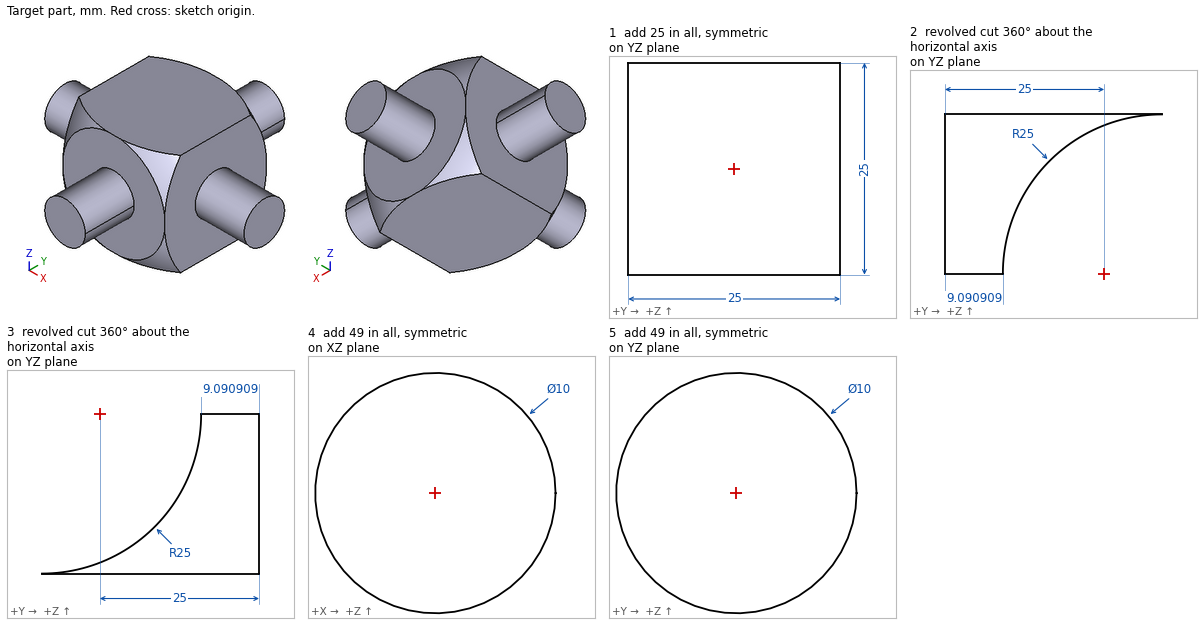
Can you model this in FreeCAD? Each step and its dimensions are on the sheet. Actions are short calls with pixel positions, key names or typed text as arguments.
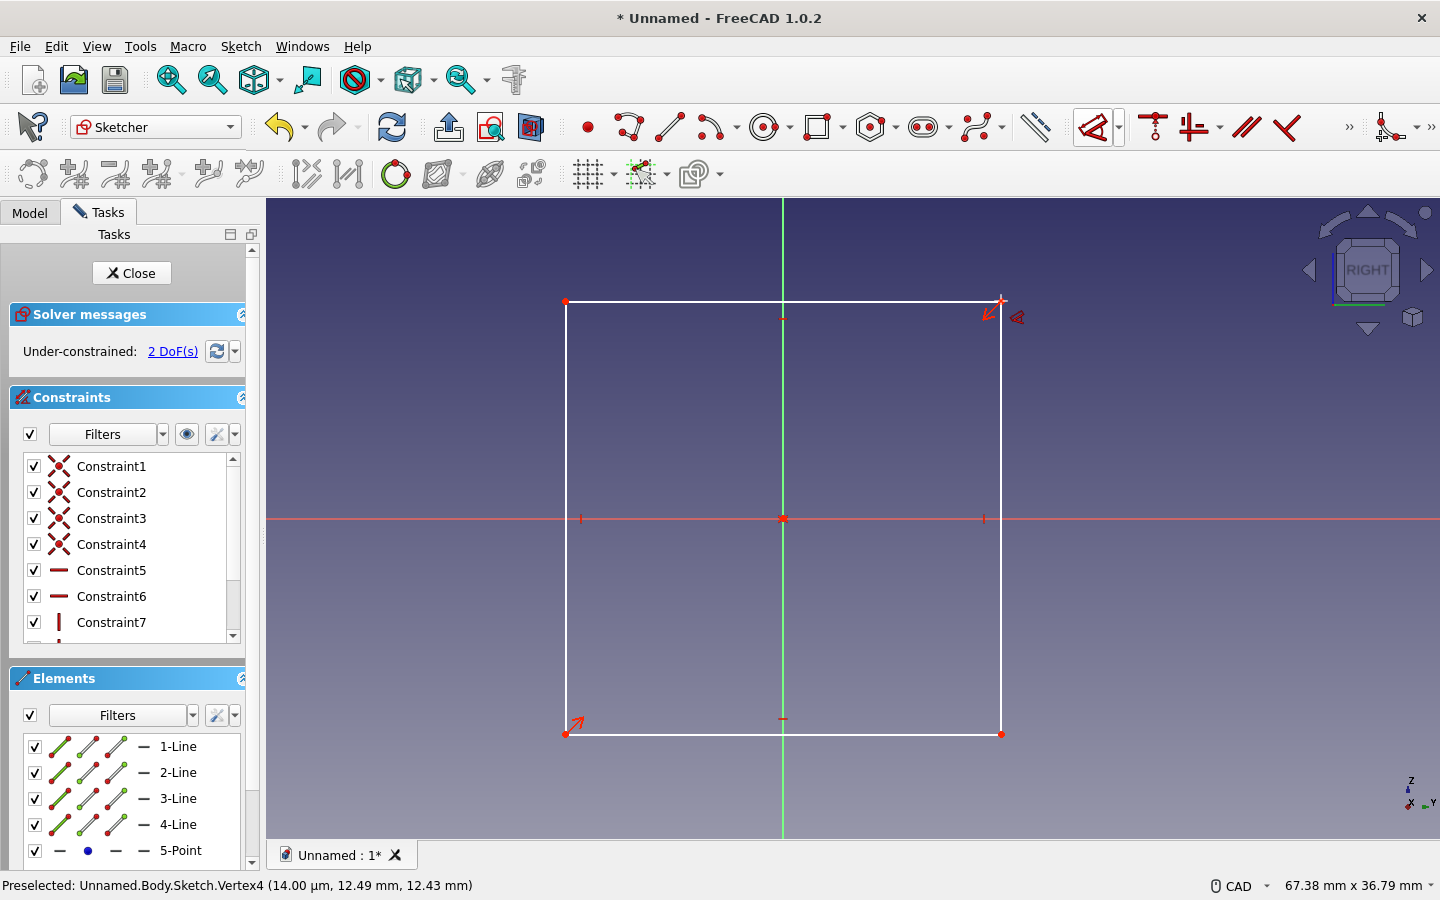
click(696, 735)
click(683, 769)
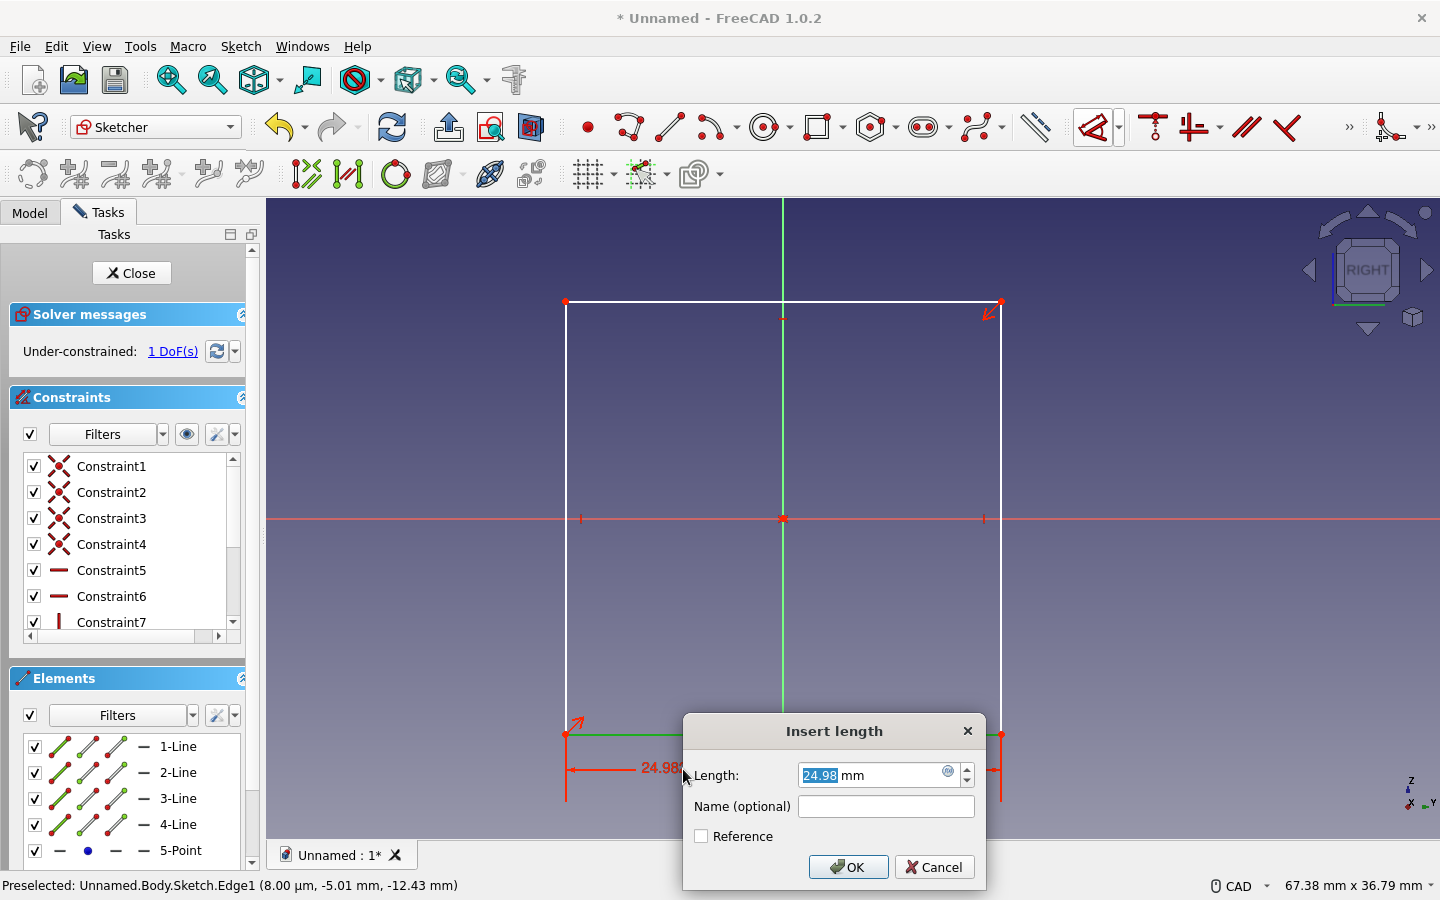
text(25)
key(Return)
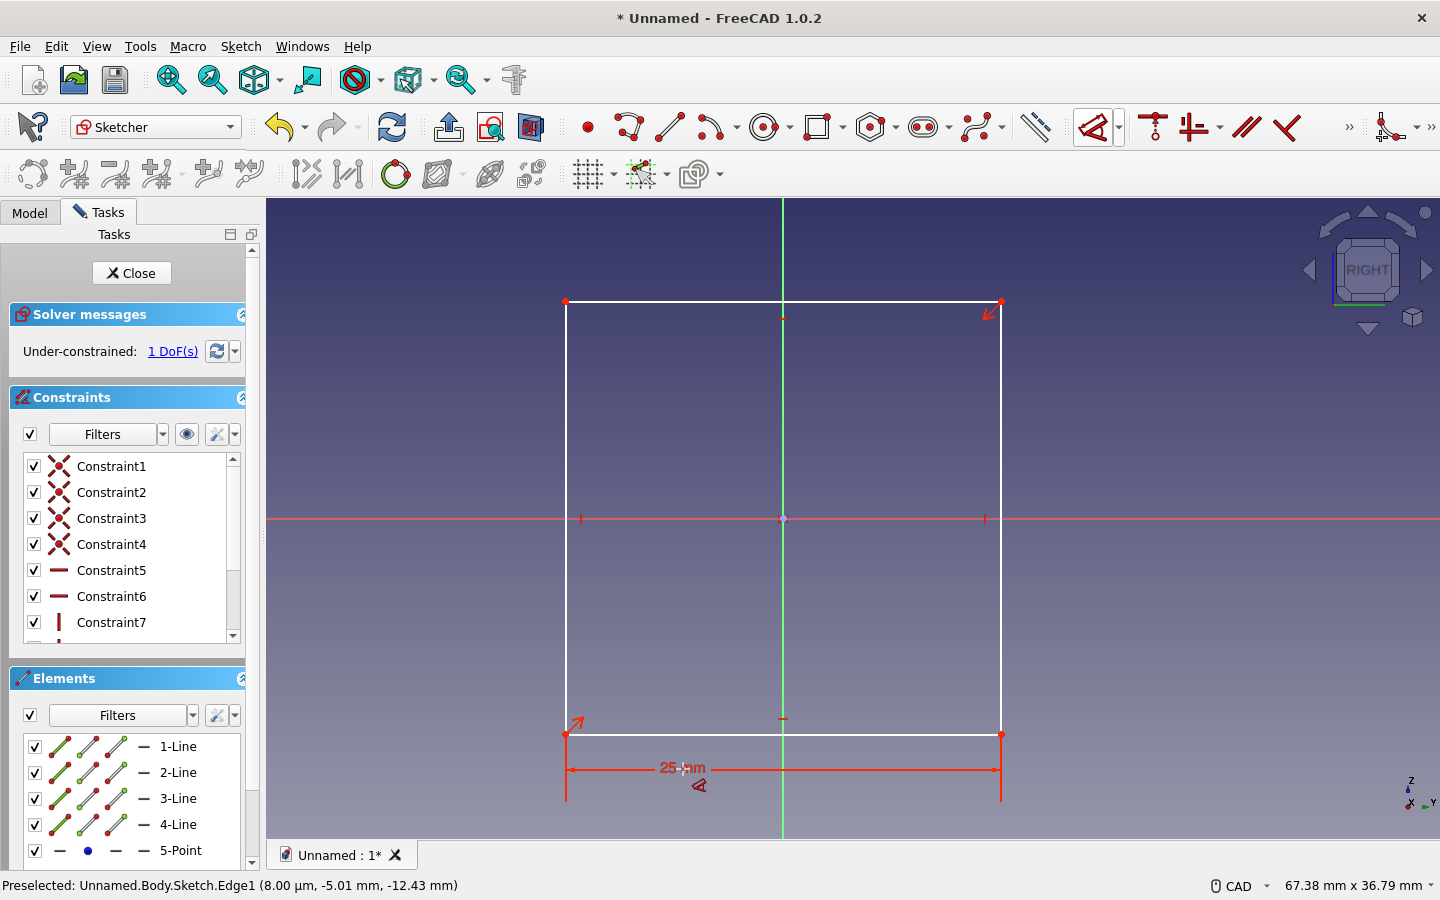
click(1001, 605)
click(1035, 419)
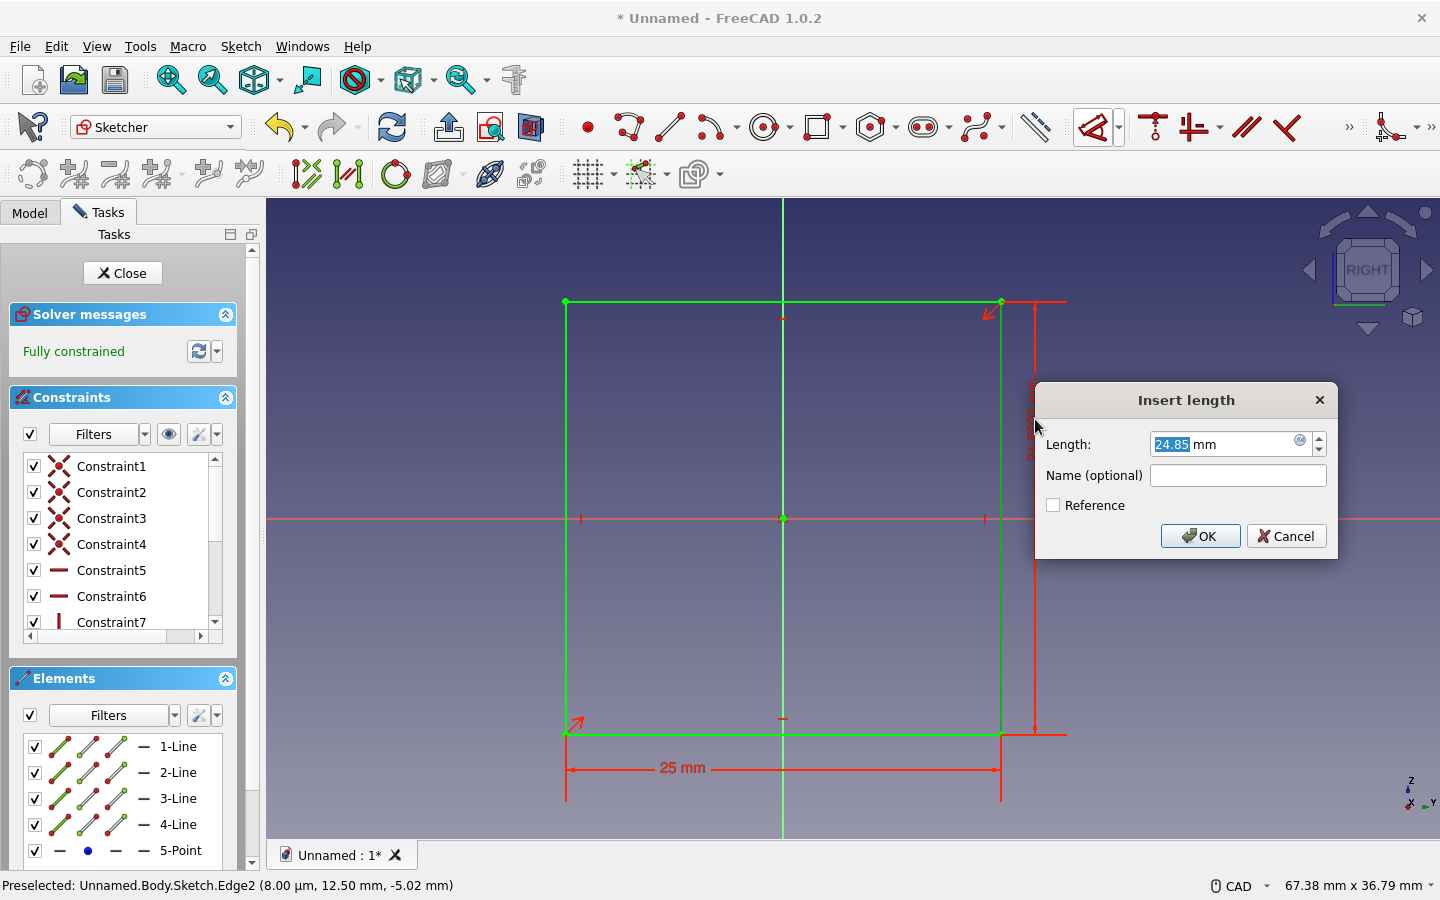
text(25)
key(Return)
key(Escape)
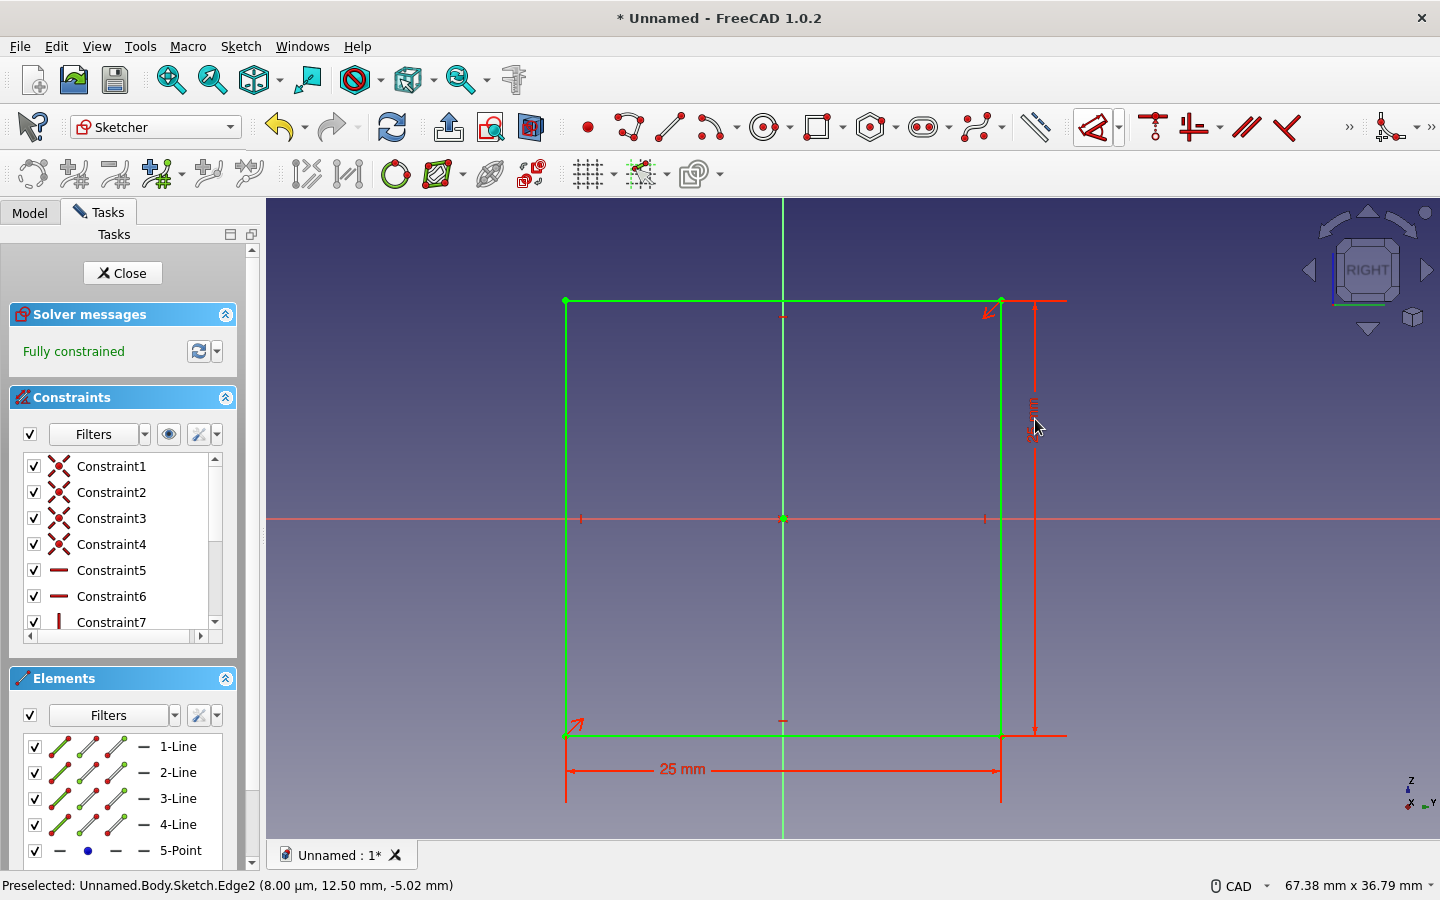
click(123, 273)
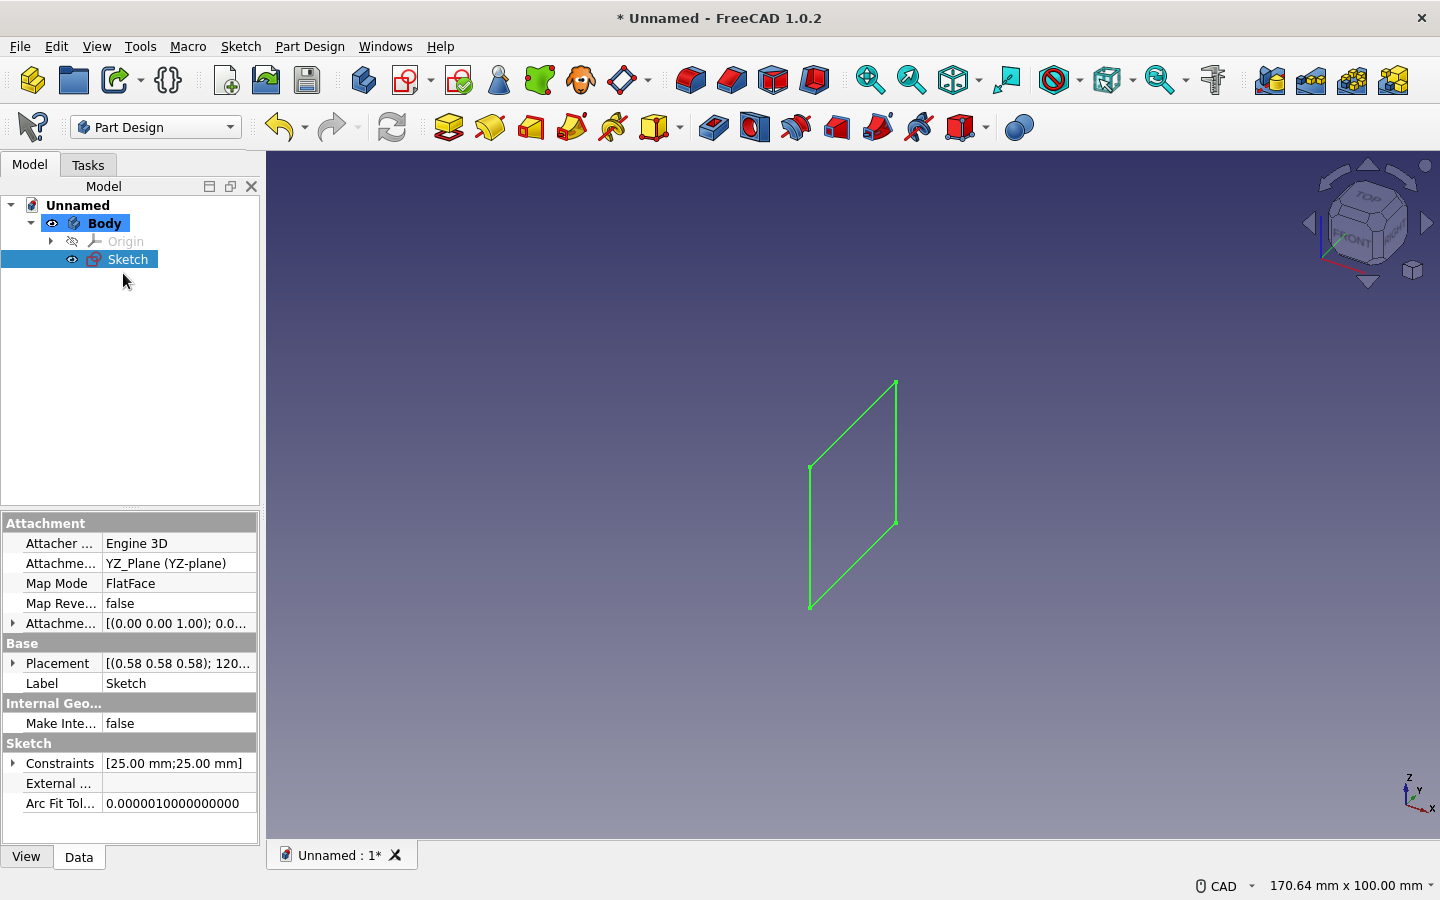
click(449, 128)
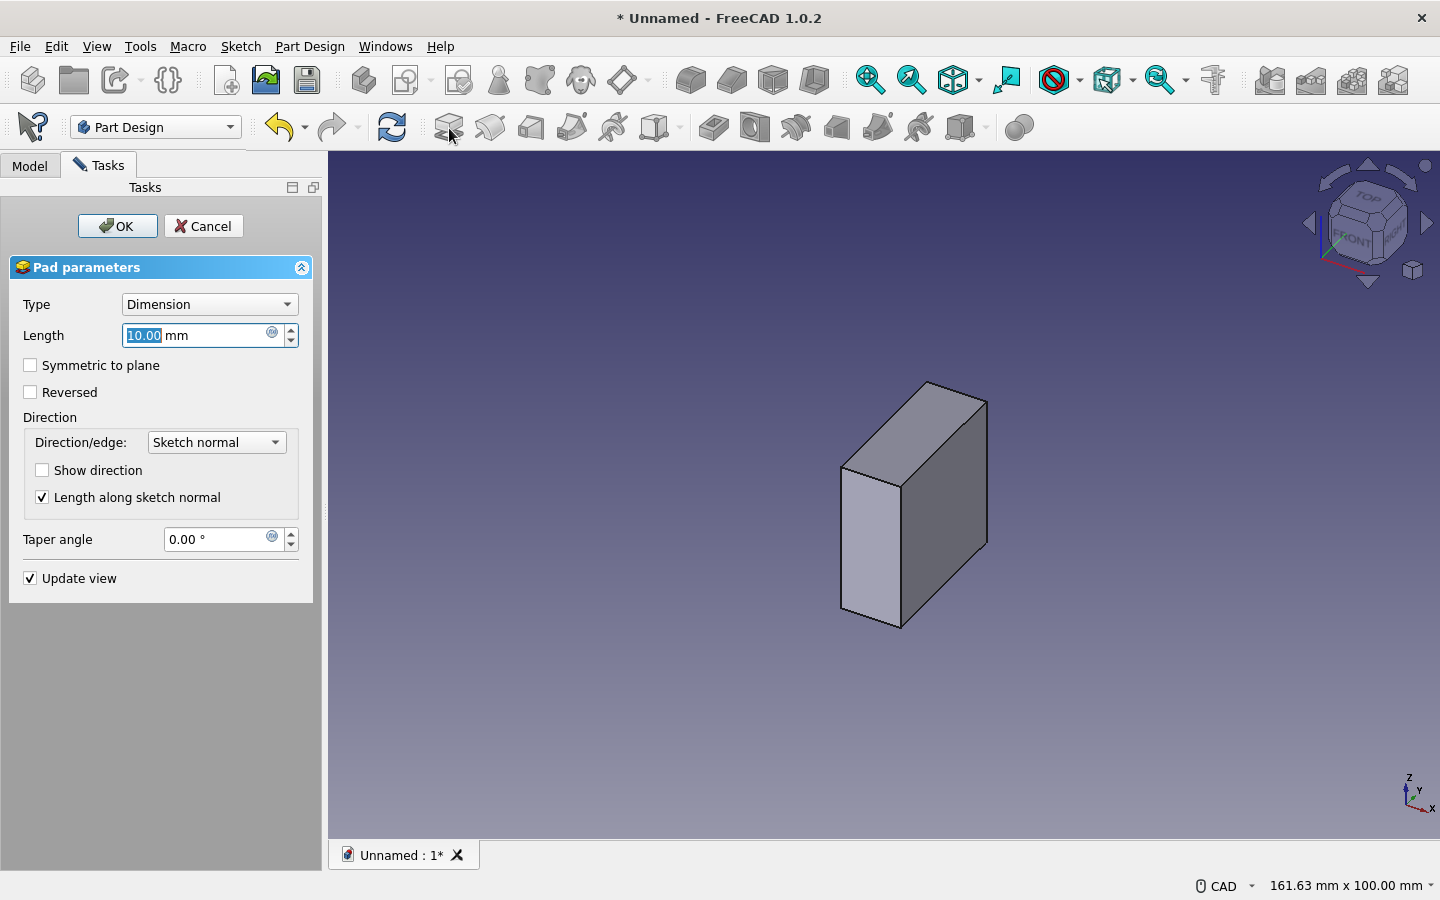
text(25)
key(Tab)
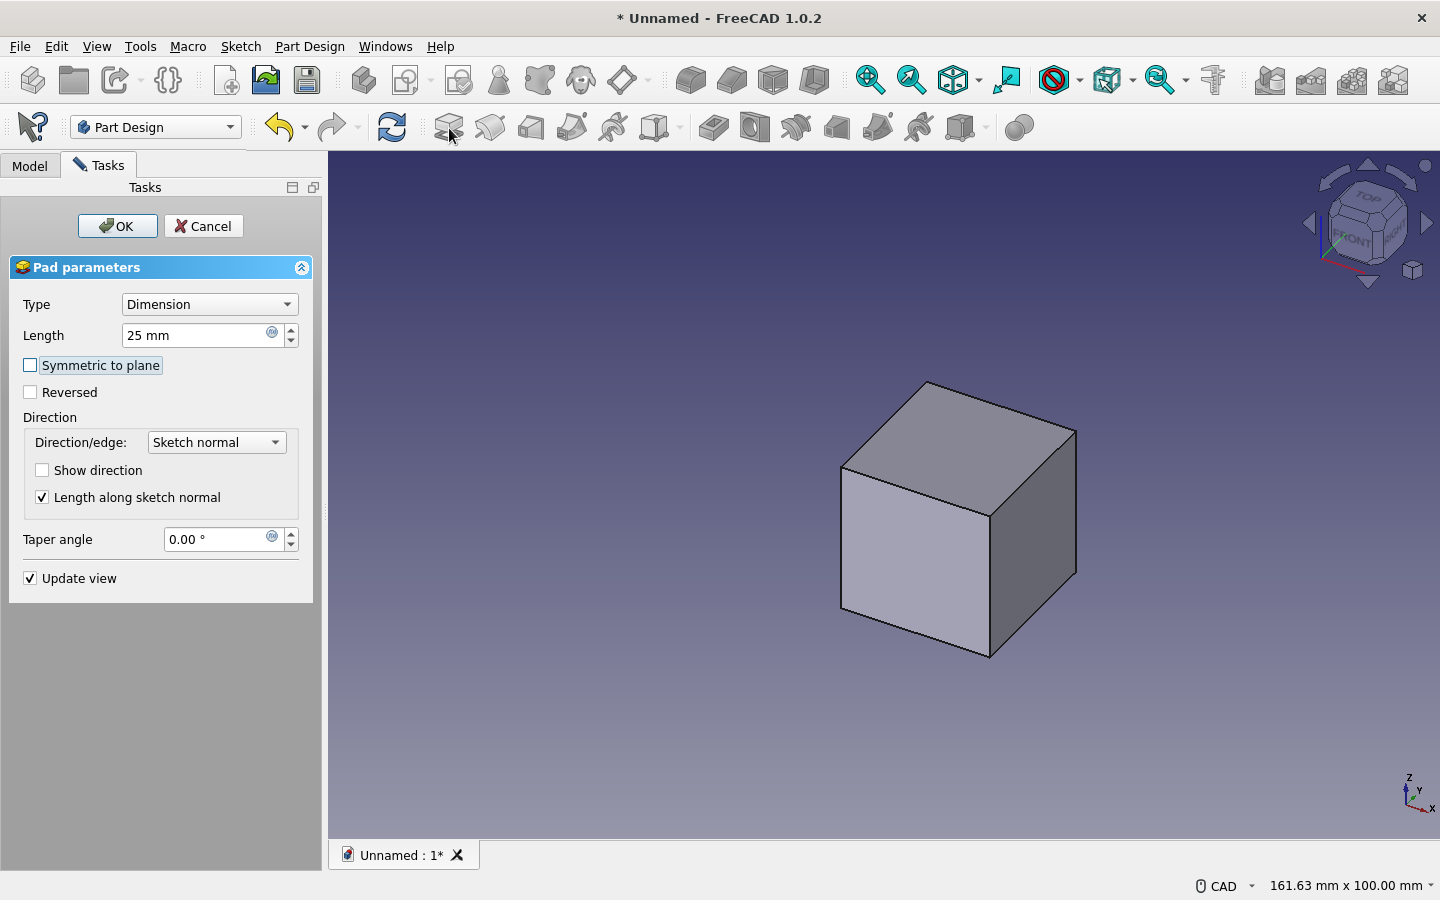
click(31, 365)